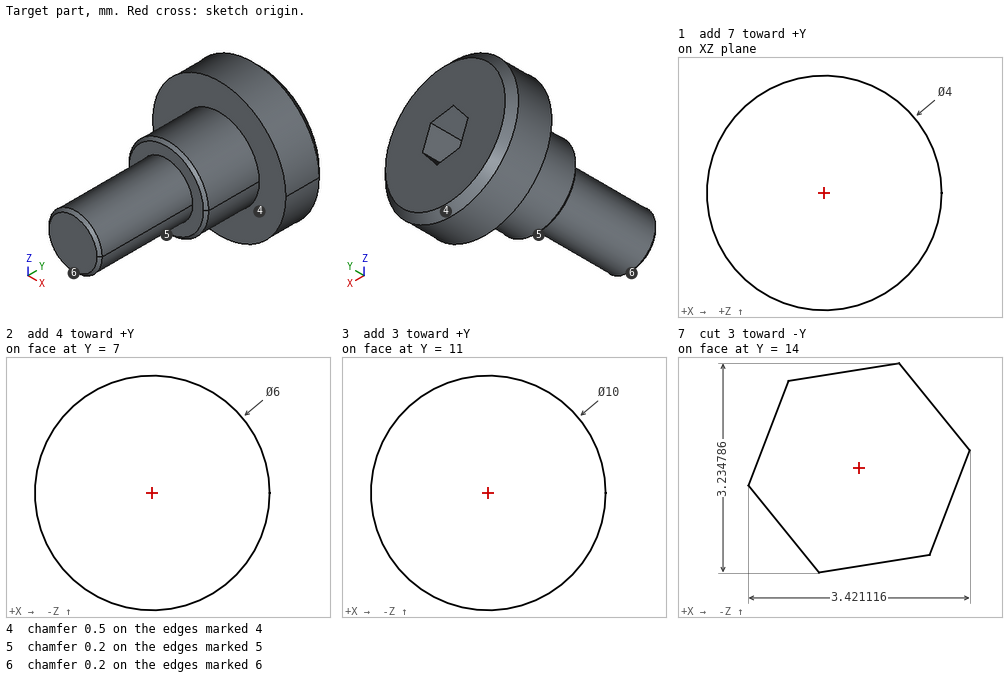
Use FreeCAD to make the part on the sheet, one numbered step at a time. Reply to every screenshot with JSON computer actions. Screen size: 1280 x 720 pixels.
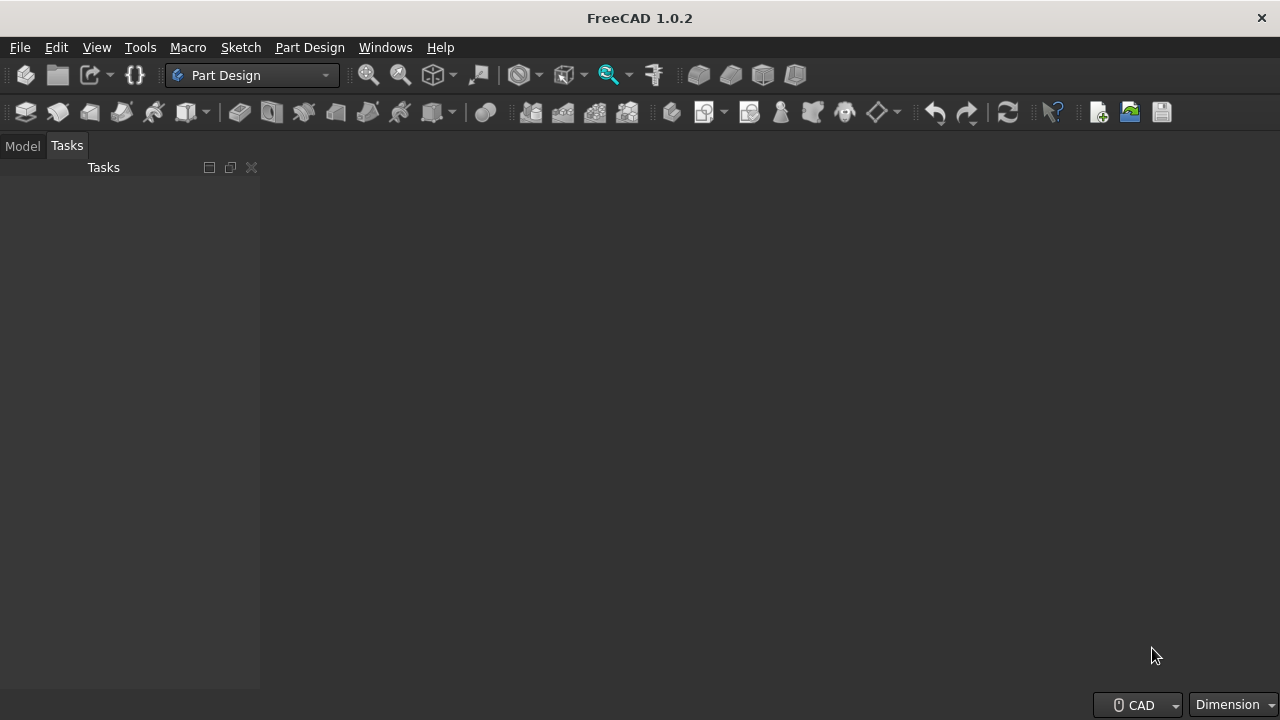
{"action": "left_click", "coordinate": [1098, 112]}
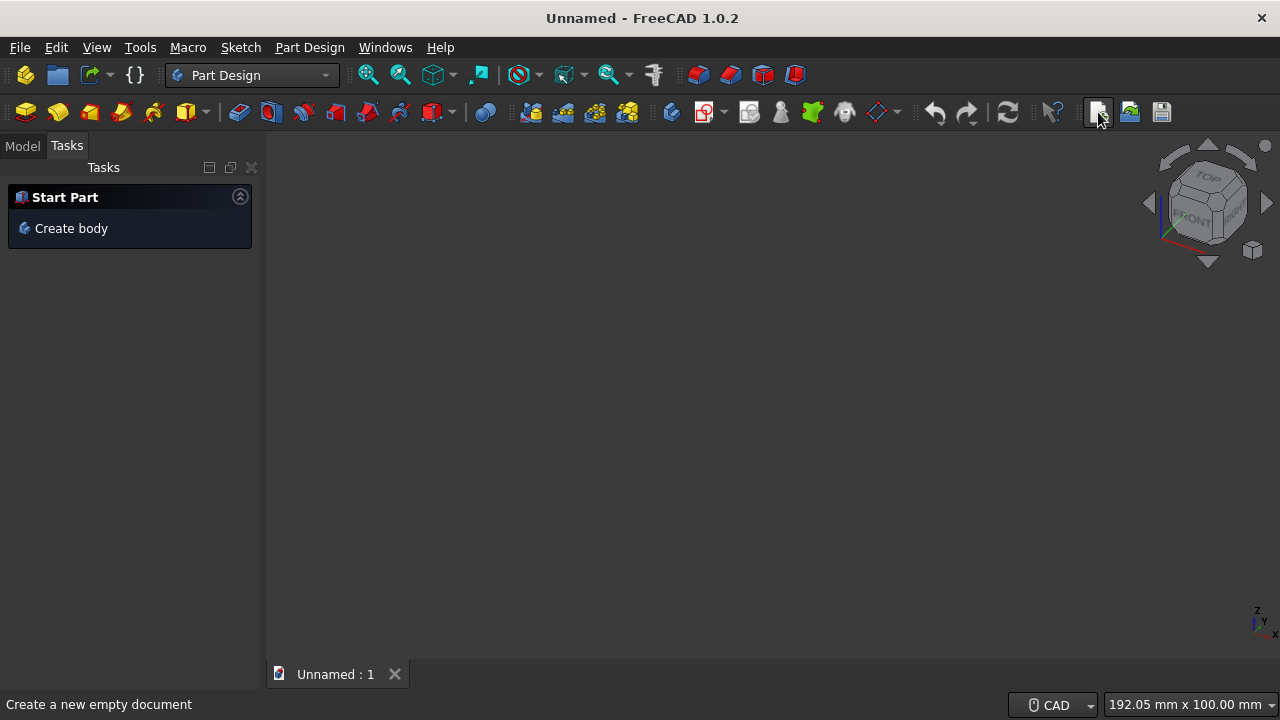
{"action": "left_click", "coordinate": [704, 112]}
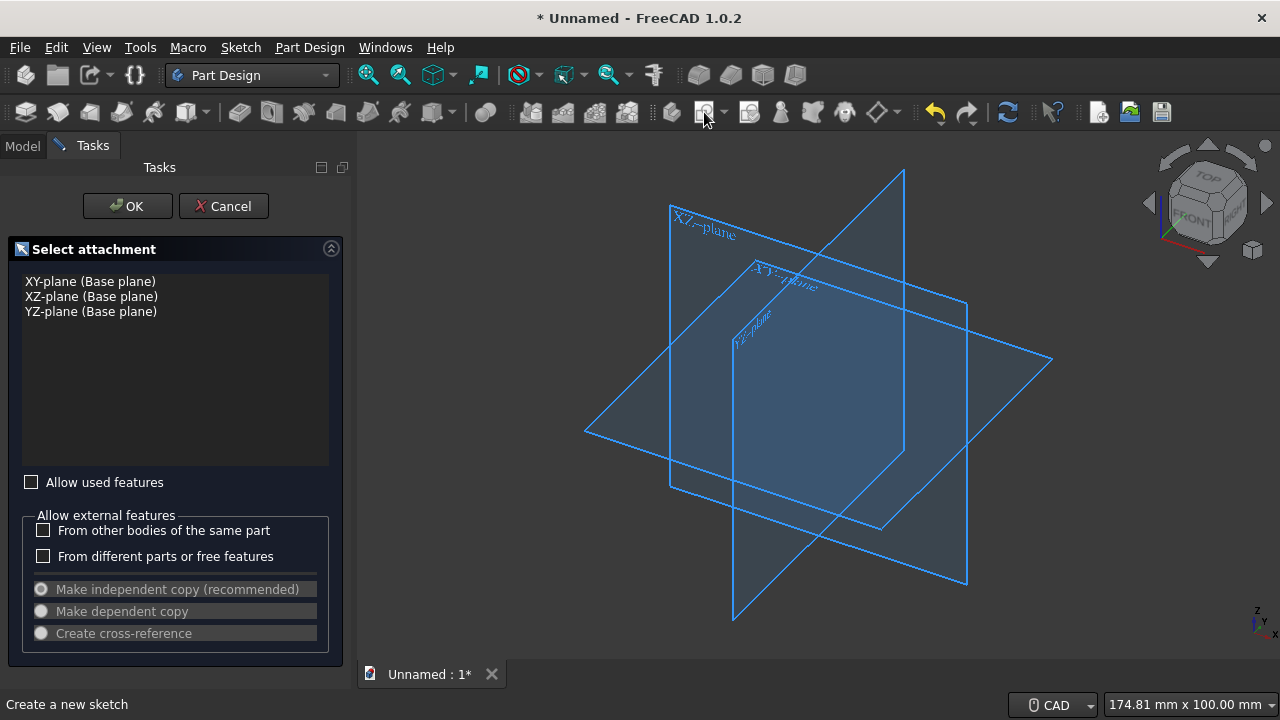
{"action": "left_click", "coordinate": [82, 296]}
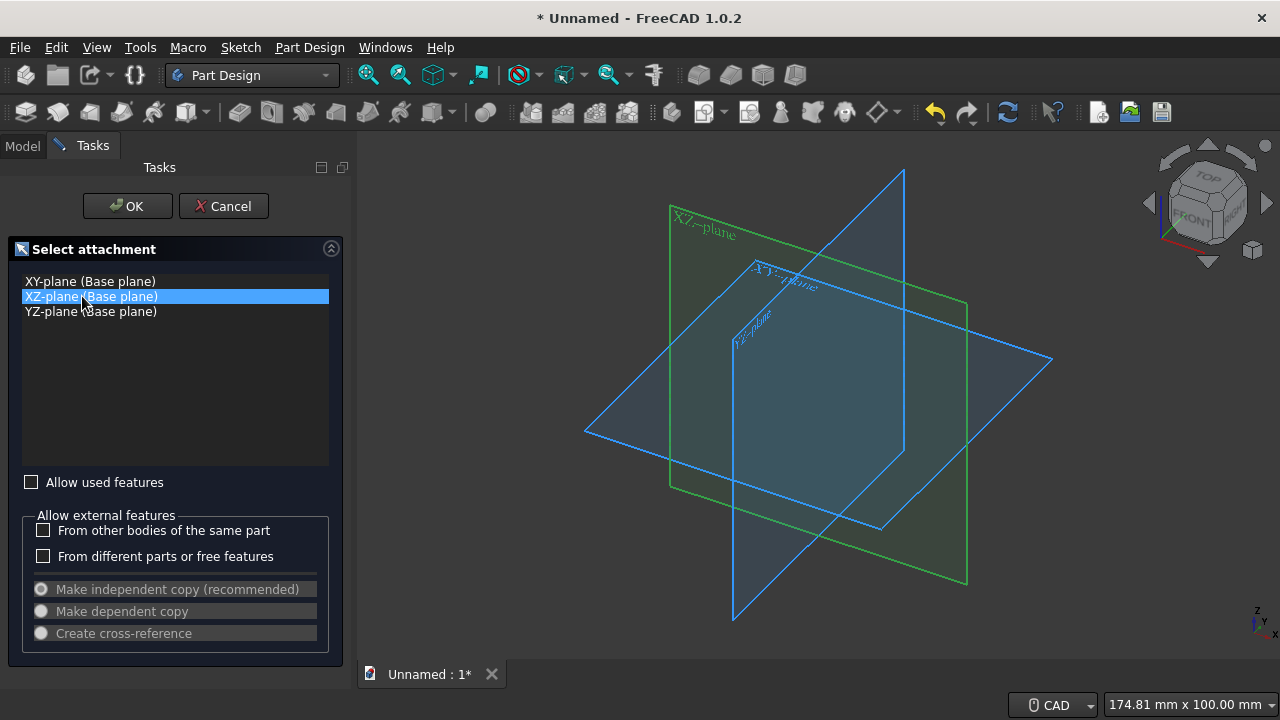
{"action": "left_click", "coordinate": [128, 206]}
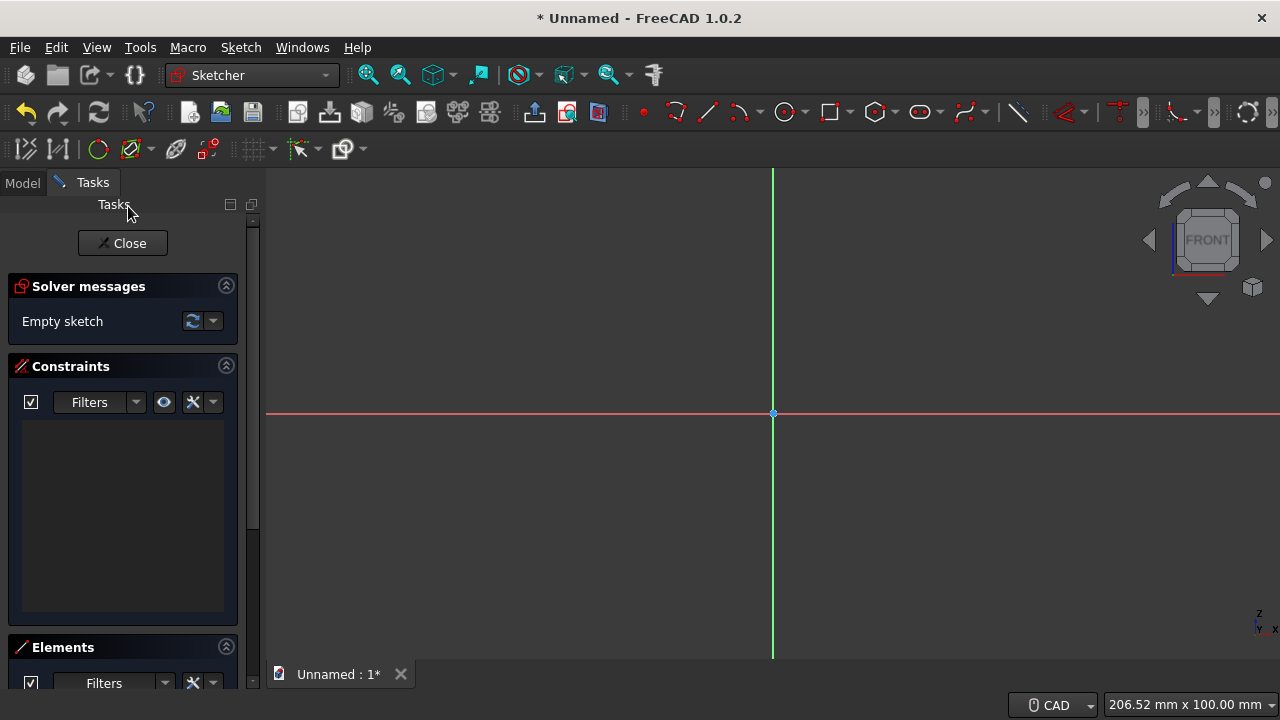
{"action": "scroll", "coordinate": [777, 414], "scroll_direction": "up", "scroll_amount": 14}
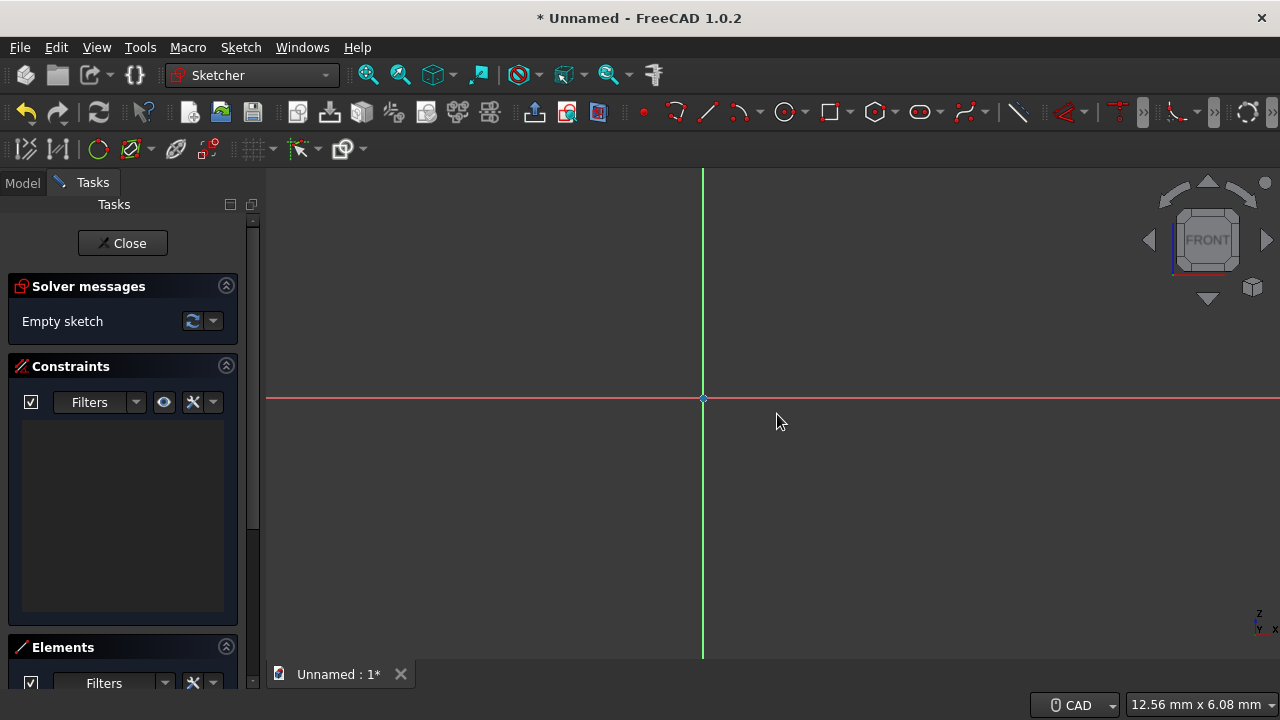
{"action": "key", "text": "g c"}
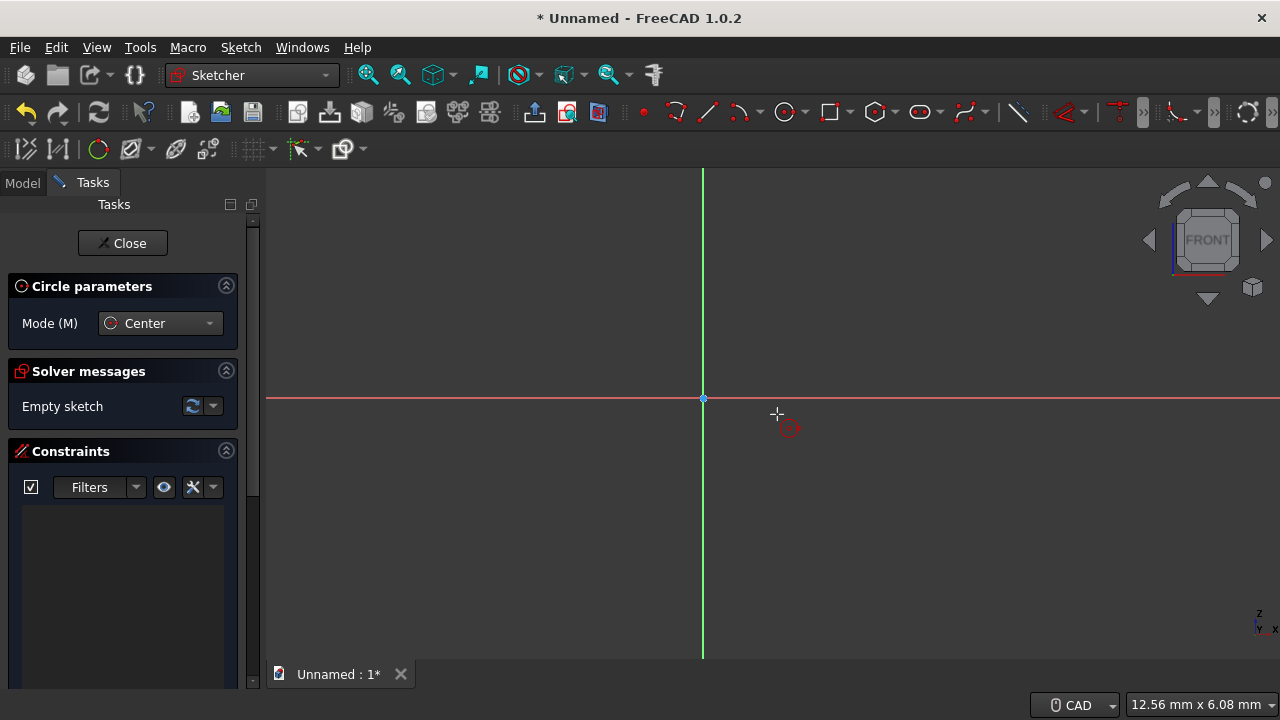
{"action": "left_click", "coordinate": [703, 398]}
{"action": "mouse_move", "coordinate": [818, 284]}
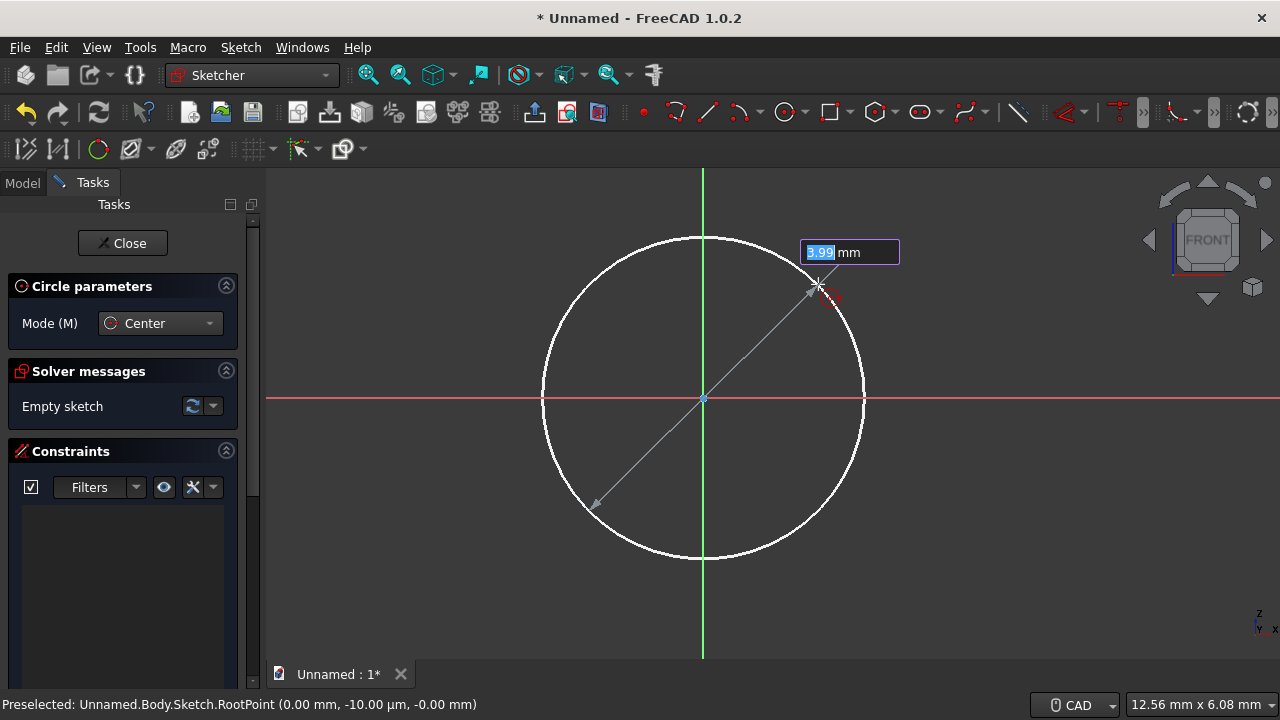
{"action": "type", "text": "4"}
{"action": "key", "text": "Return"}
{"action": "key", "text": "Escape"}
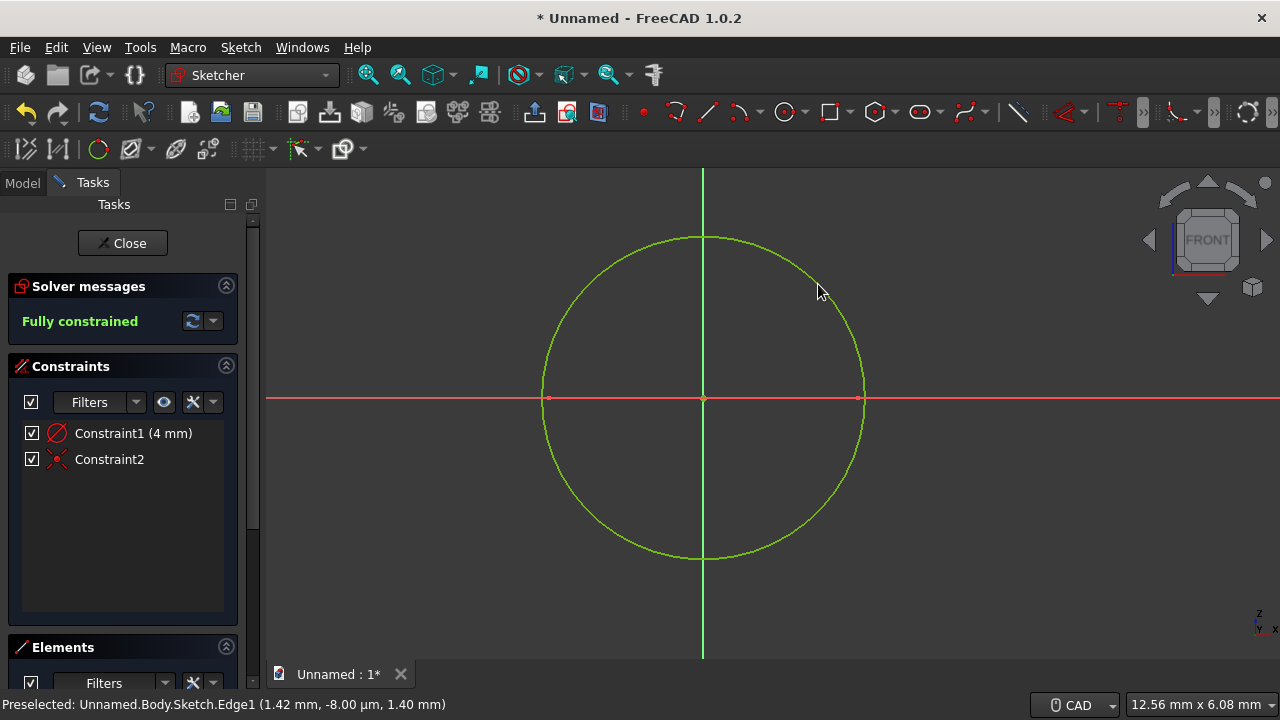
{"action": "left_click", "coordinate": [123, 243]}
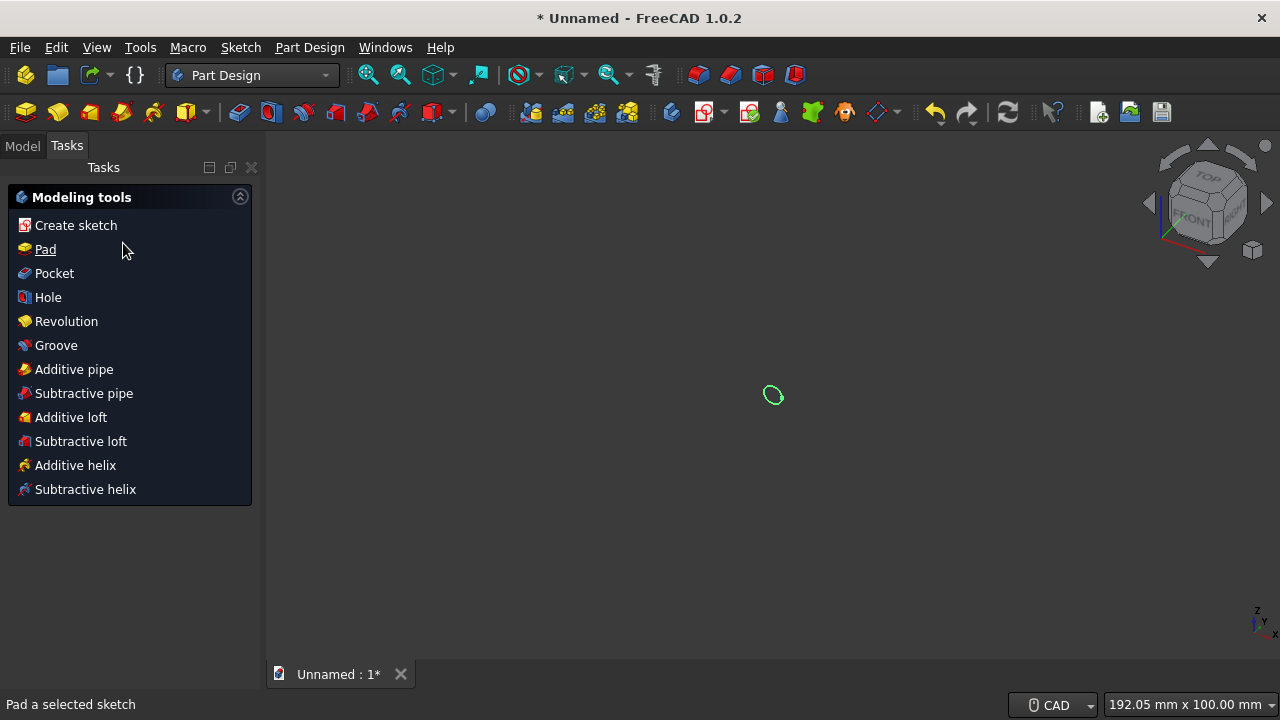
{"action": "left_click", "coordinate": [26, 112]}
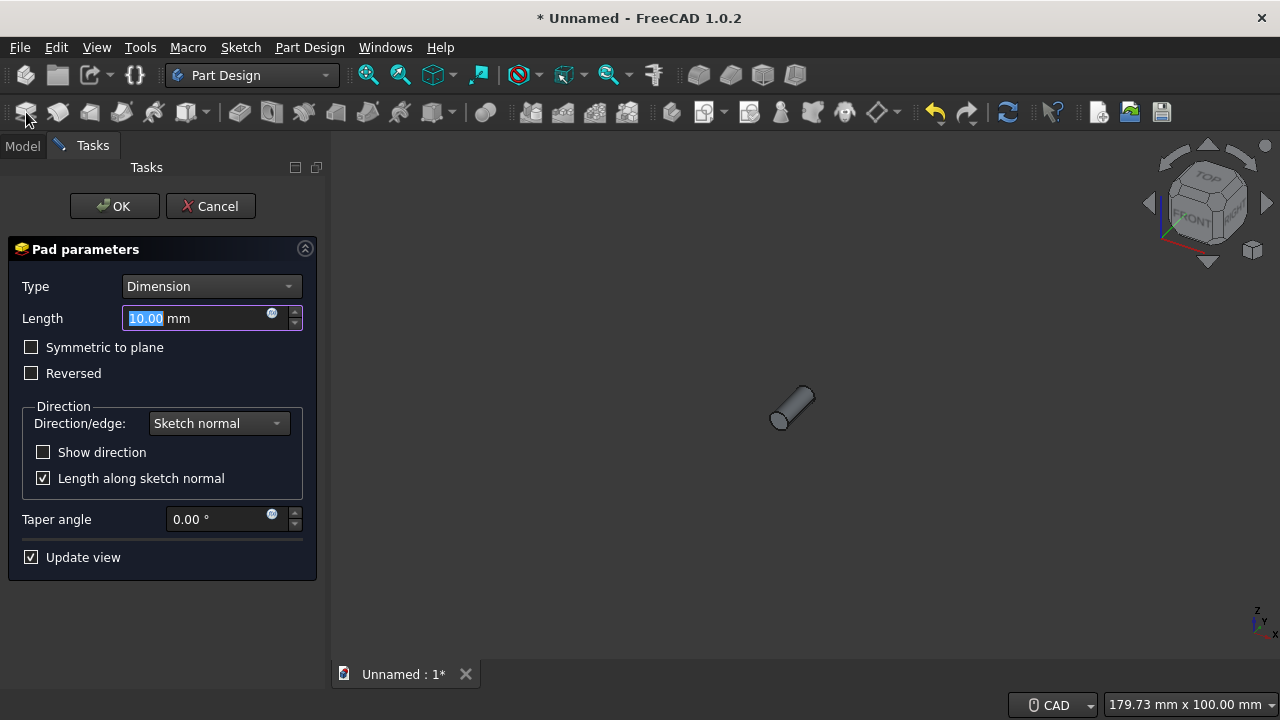
{"action": "type", "text": "7"}
{"action": "key", "text": "Tab"}